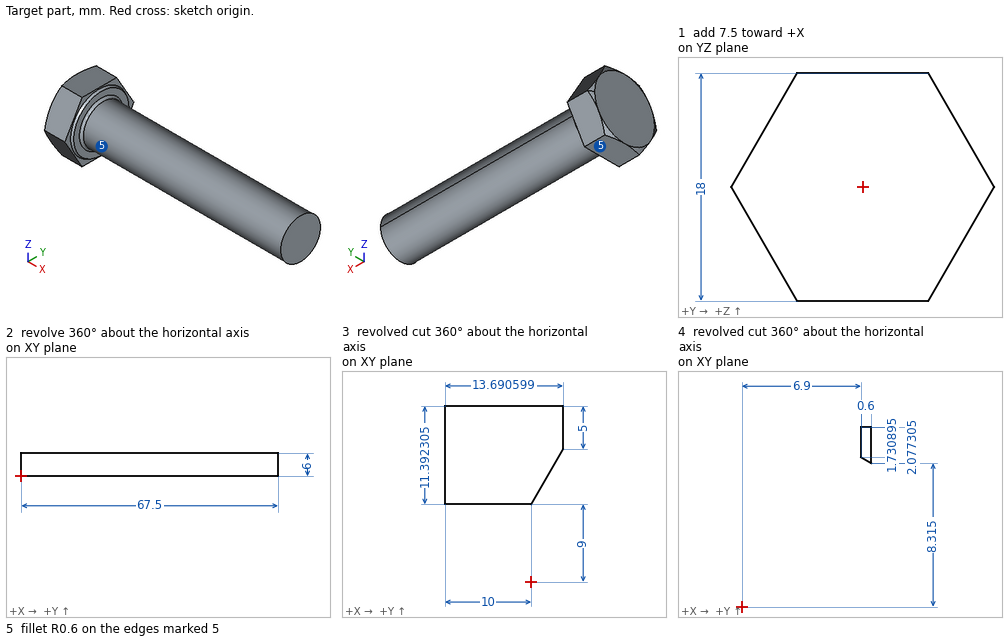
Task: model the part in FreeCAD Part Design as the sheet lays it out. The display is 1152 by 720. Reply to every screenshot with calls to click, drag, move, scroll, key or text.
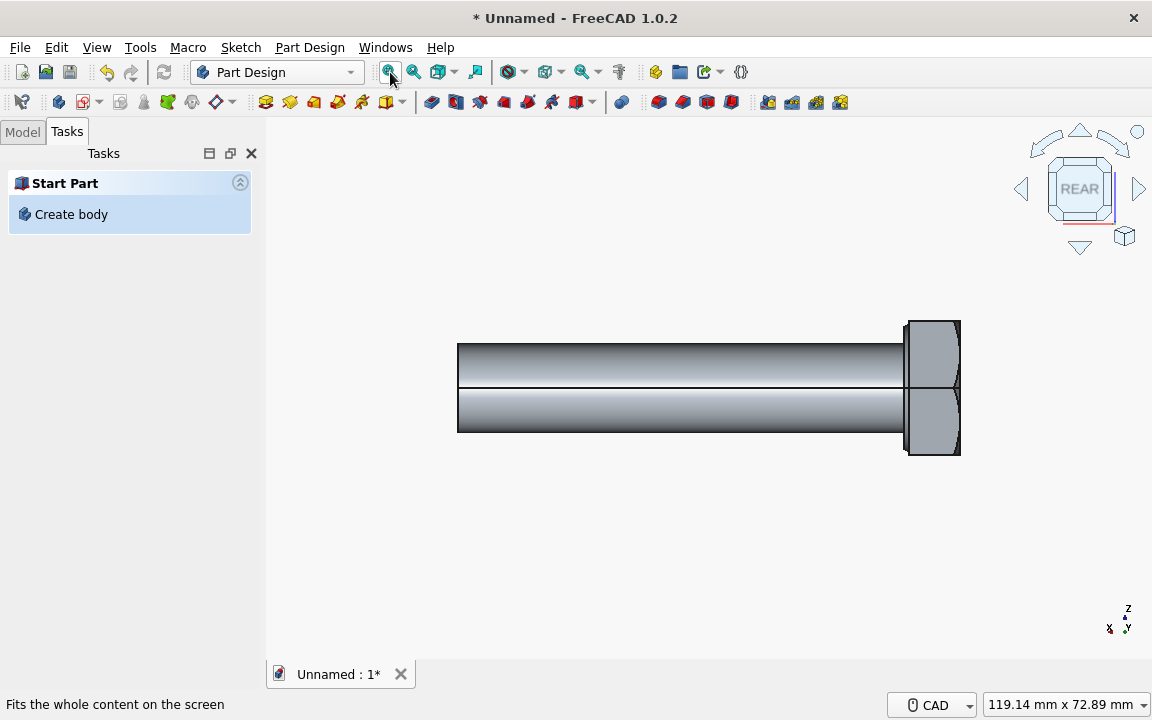
key(6)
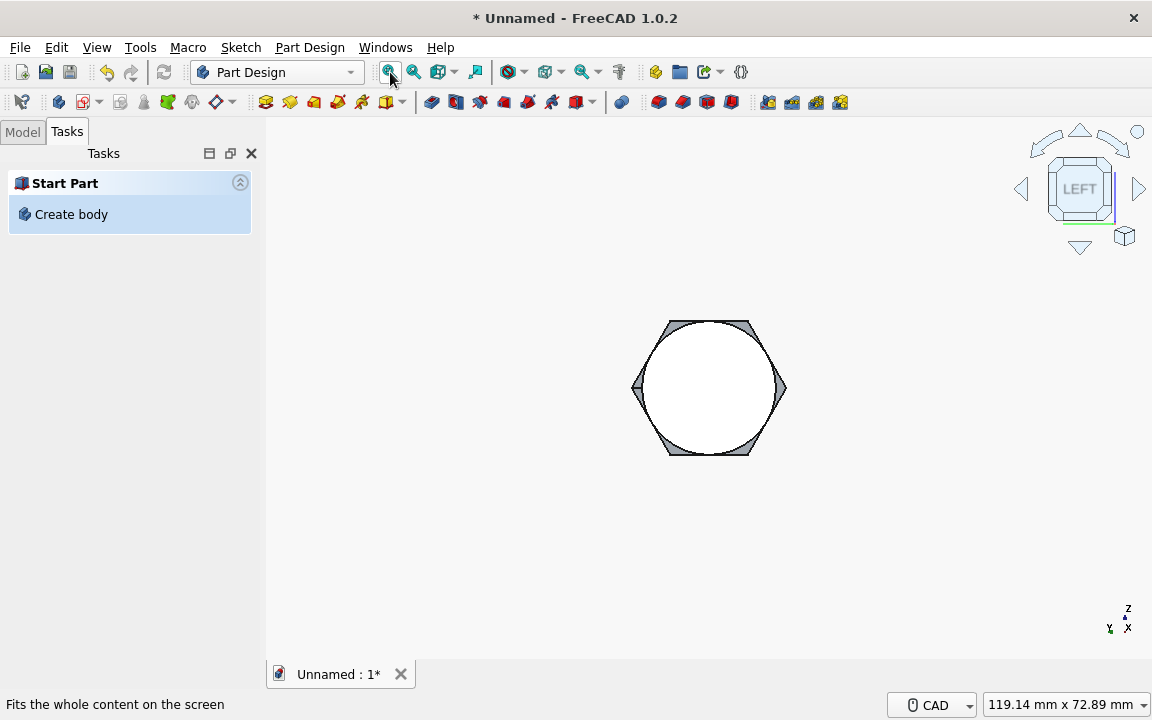
click(390, 72)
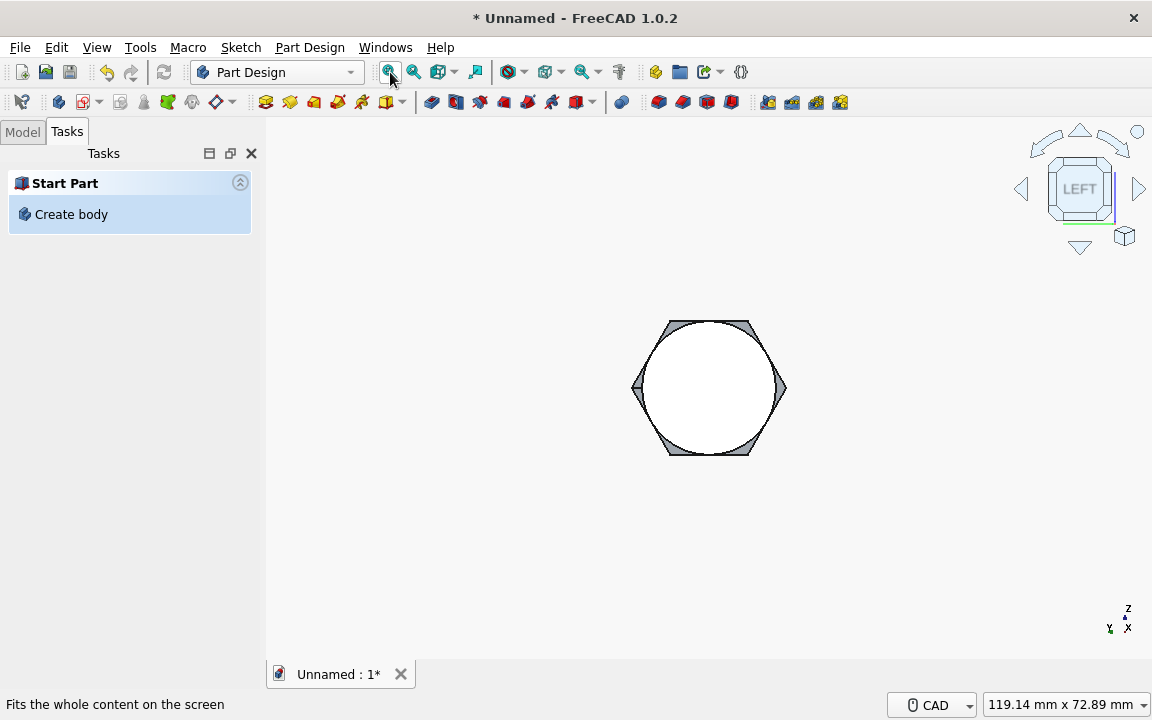
key(v)
key(3)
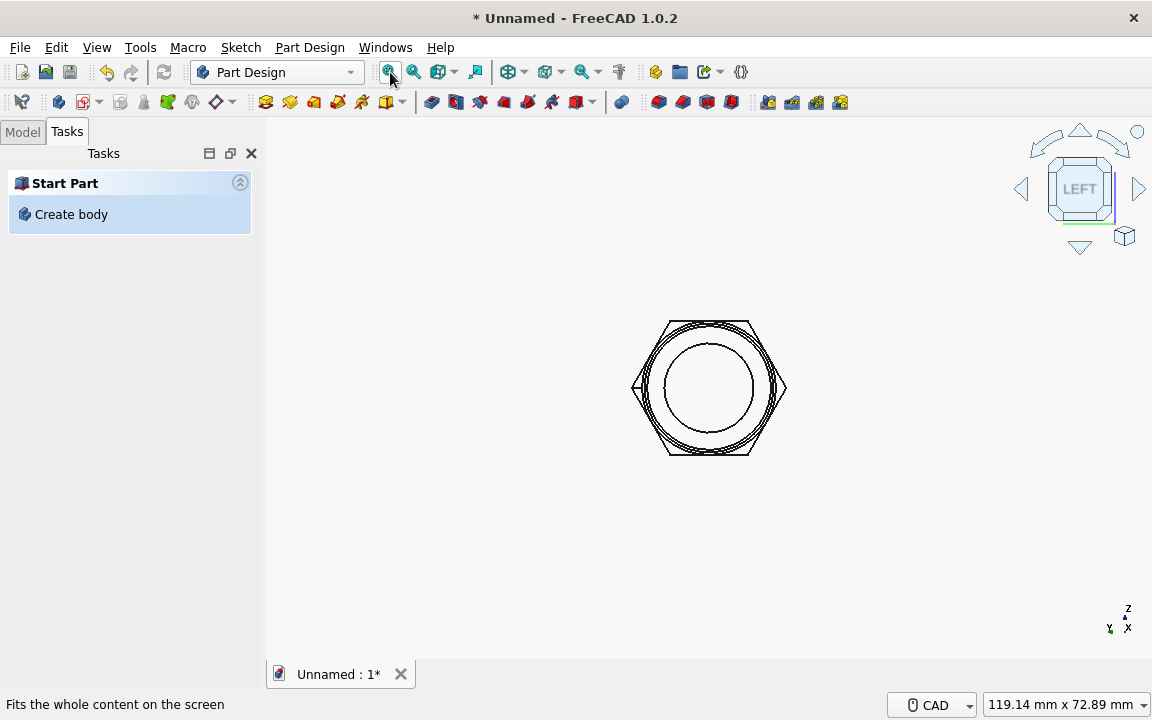
key(0)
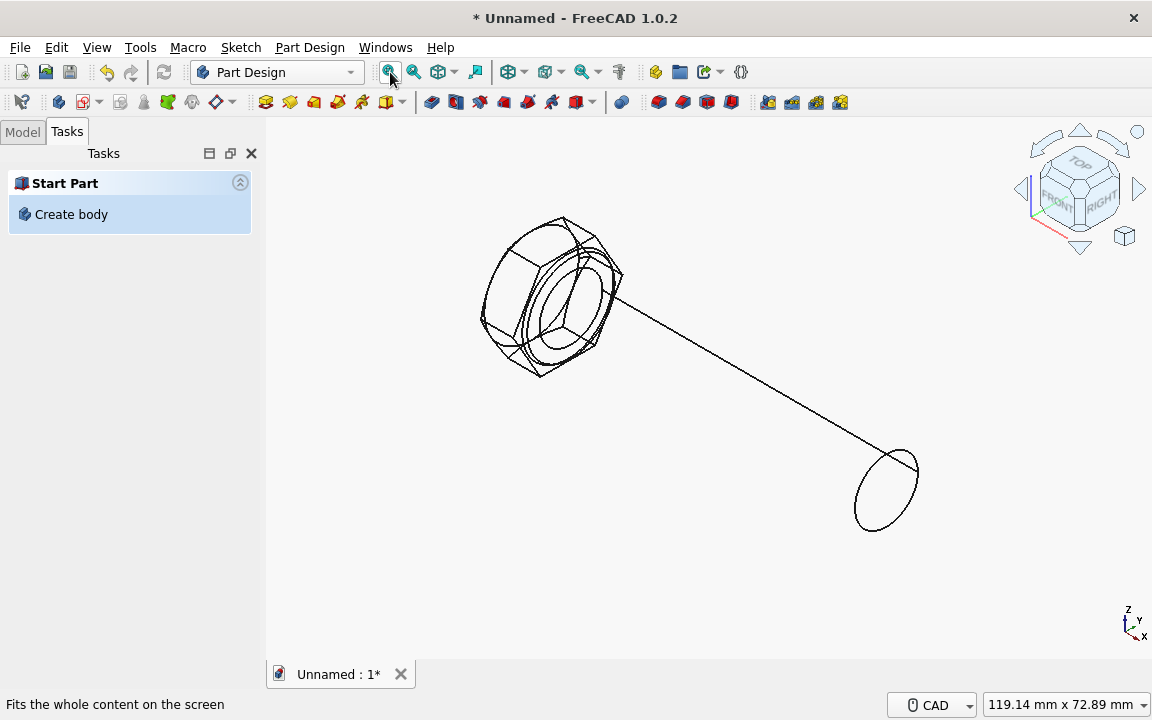
click(539, 326)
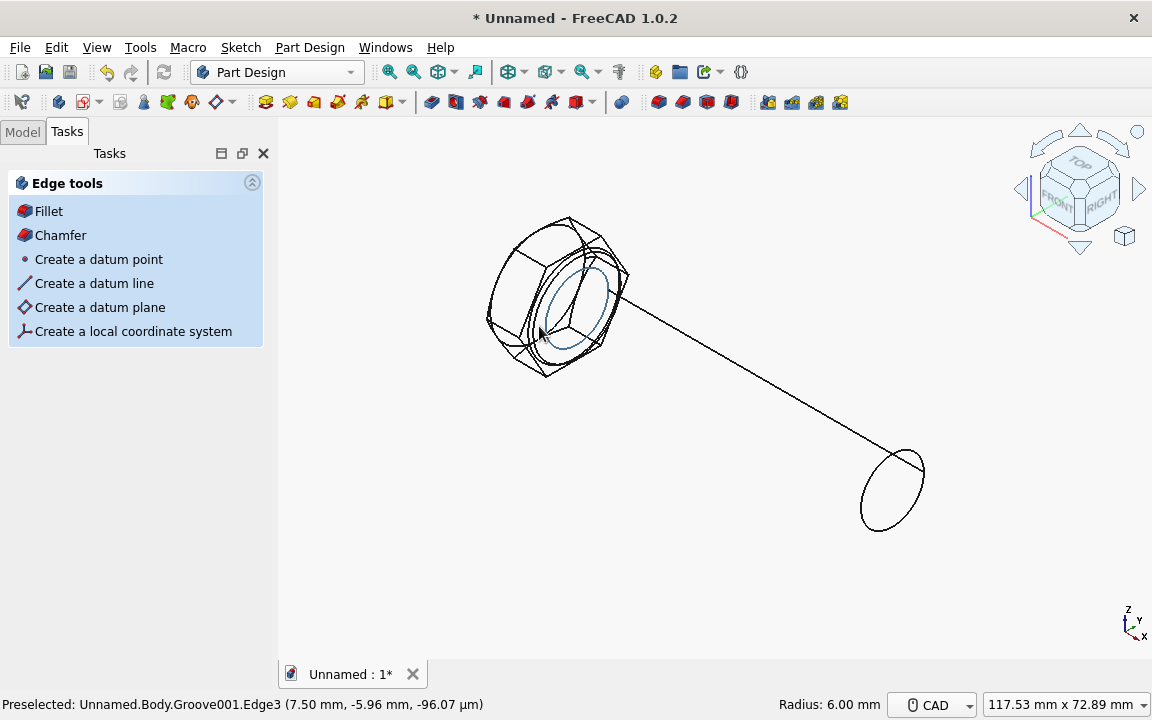
key(v)
key(1)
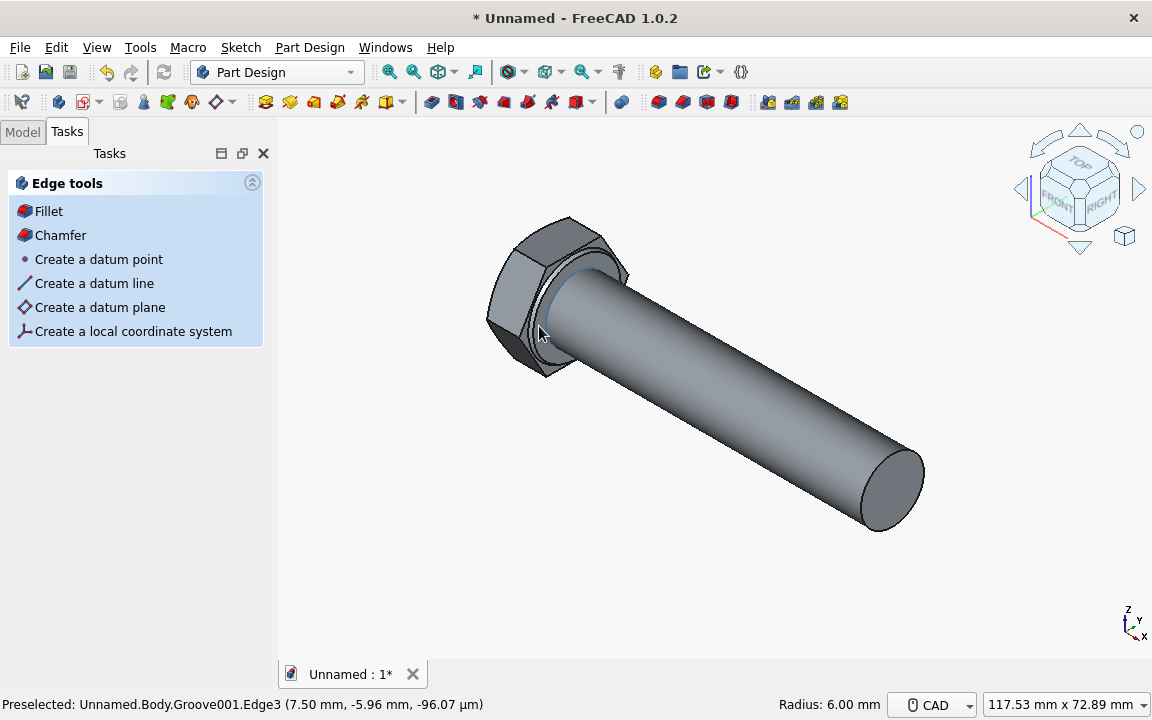
click(660, 102)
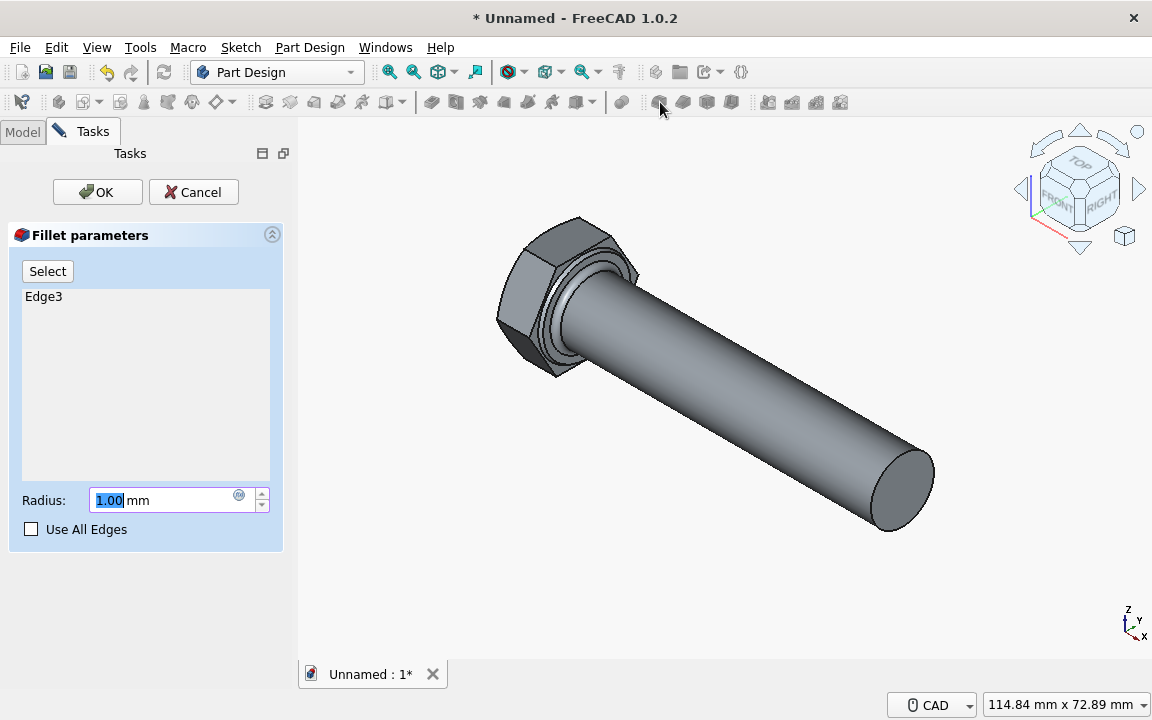
text(0.6)
key(Tab)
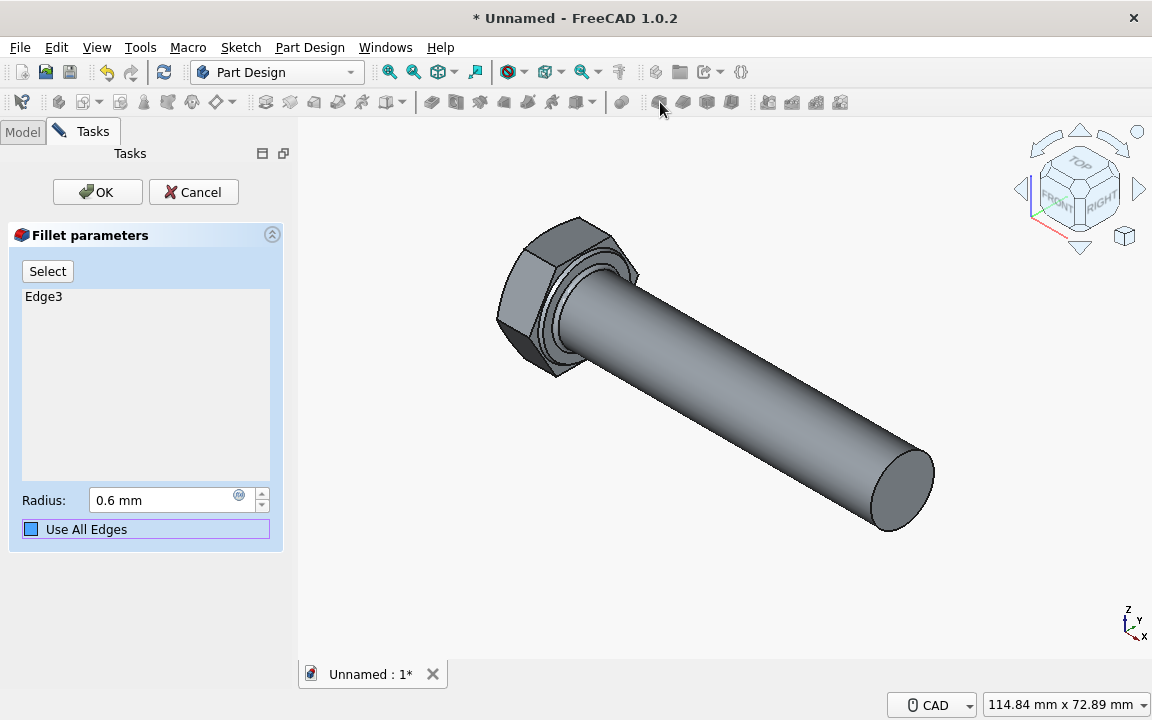
click(98, 192)